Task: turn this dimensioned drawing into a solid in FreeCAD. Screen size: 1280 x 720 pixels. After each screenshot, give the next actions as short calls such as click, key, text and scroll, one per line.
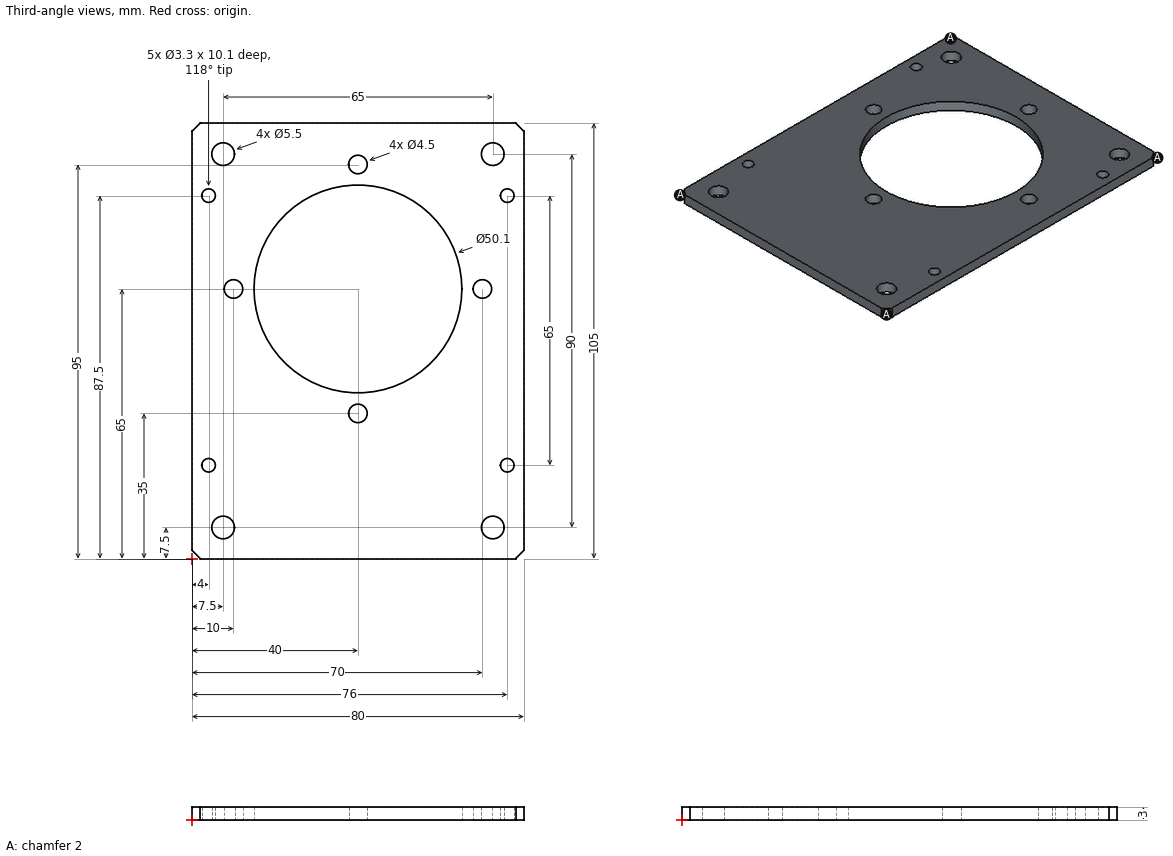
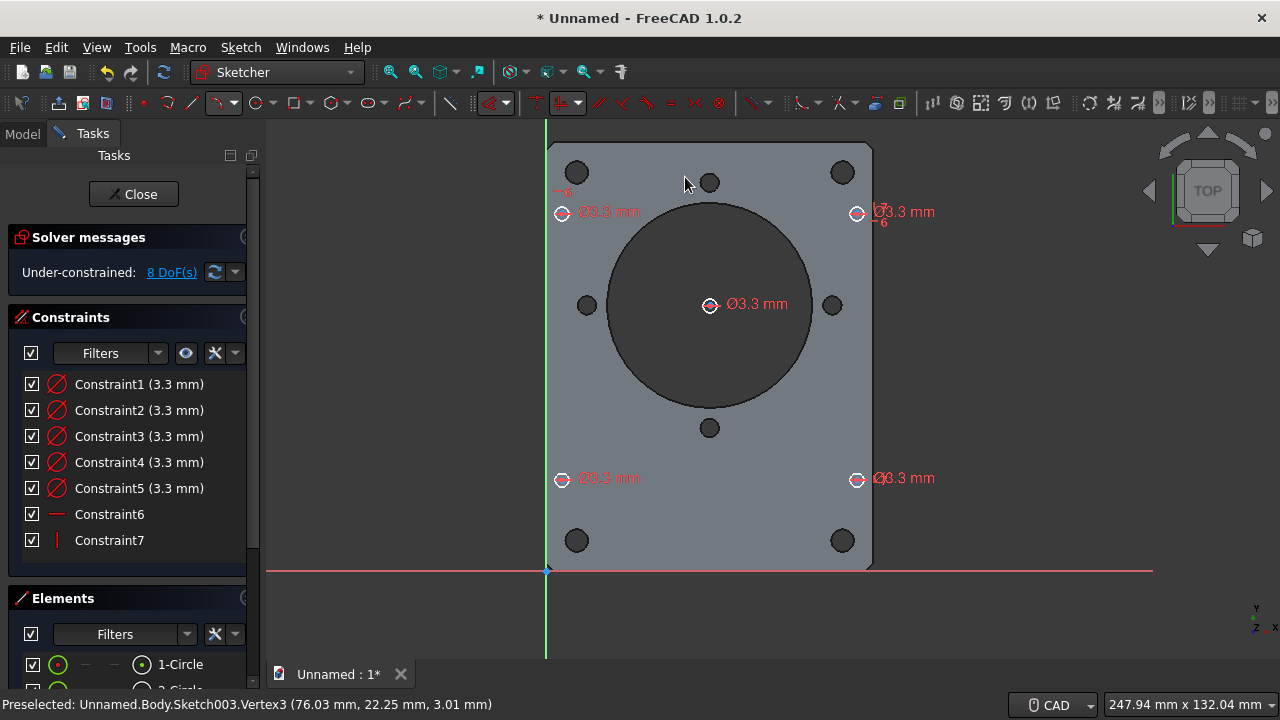
click(562, 214)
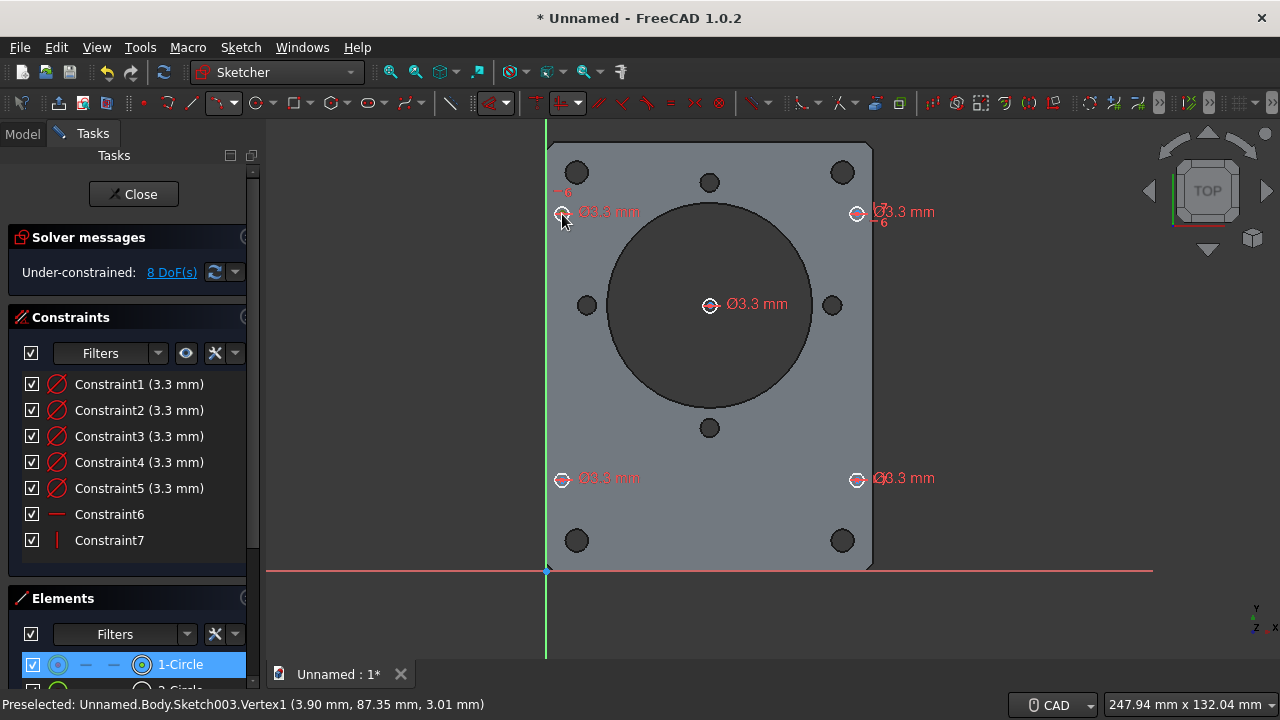
click(562, 480)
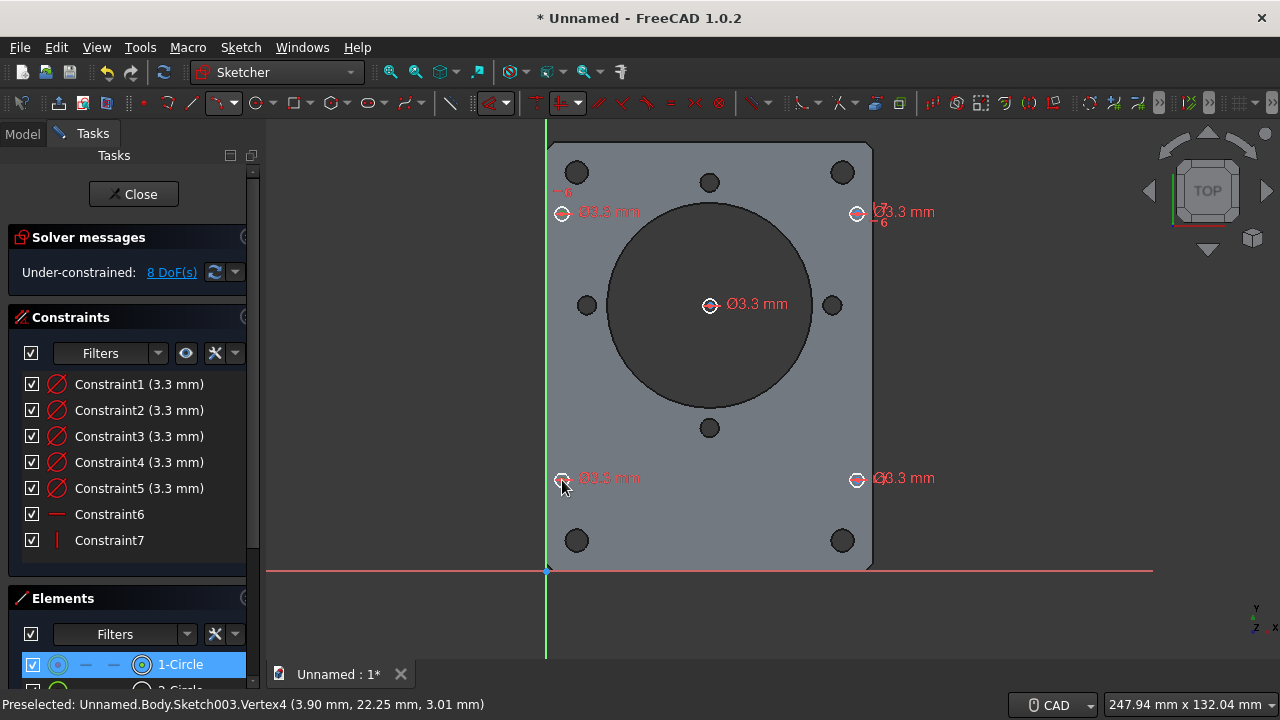
click(580, 104)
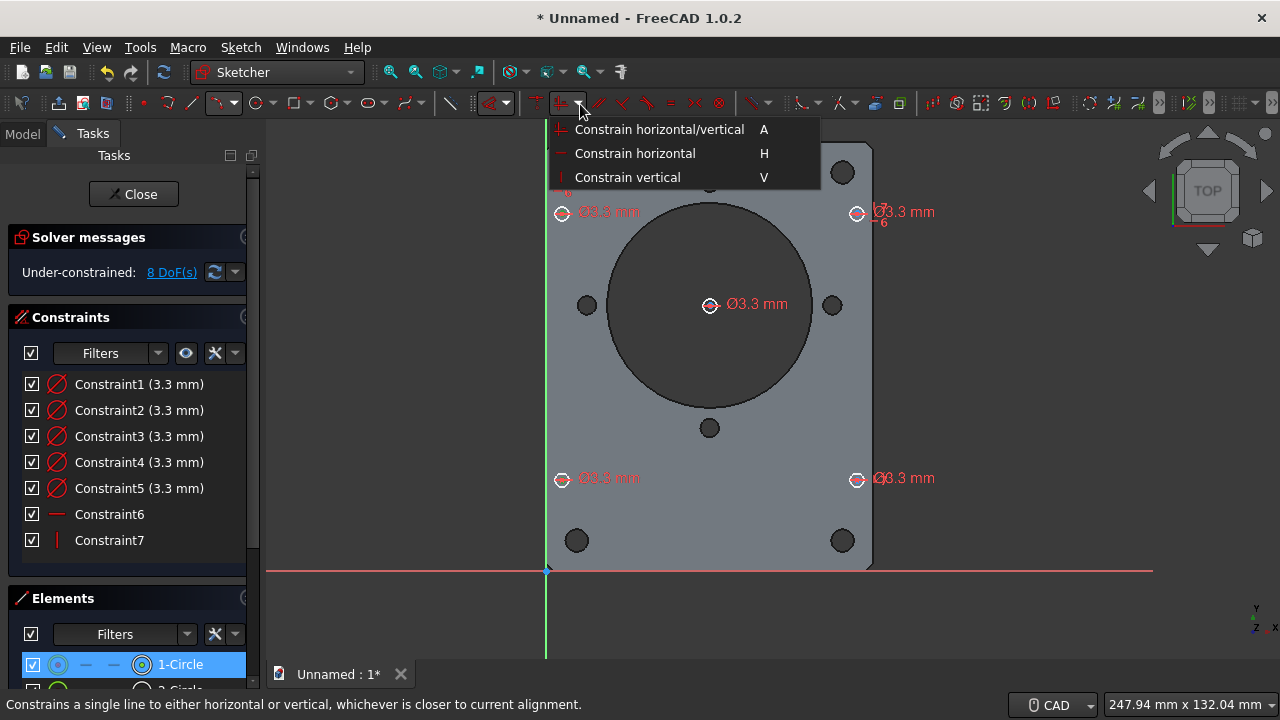
click(685, 177)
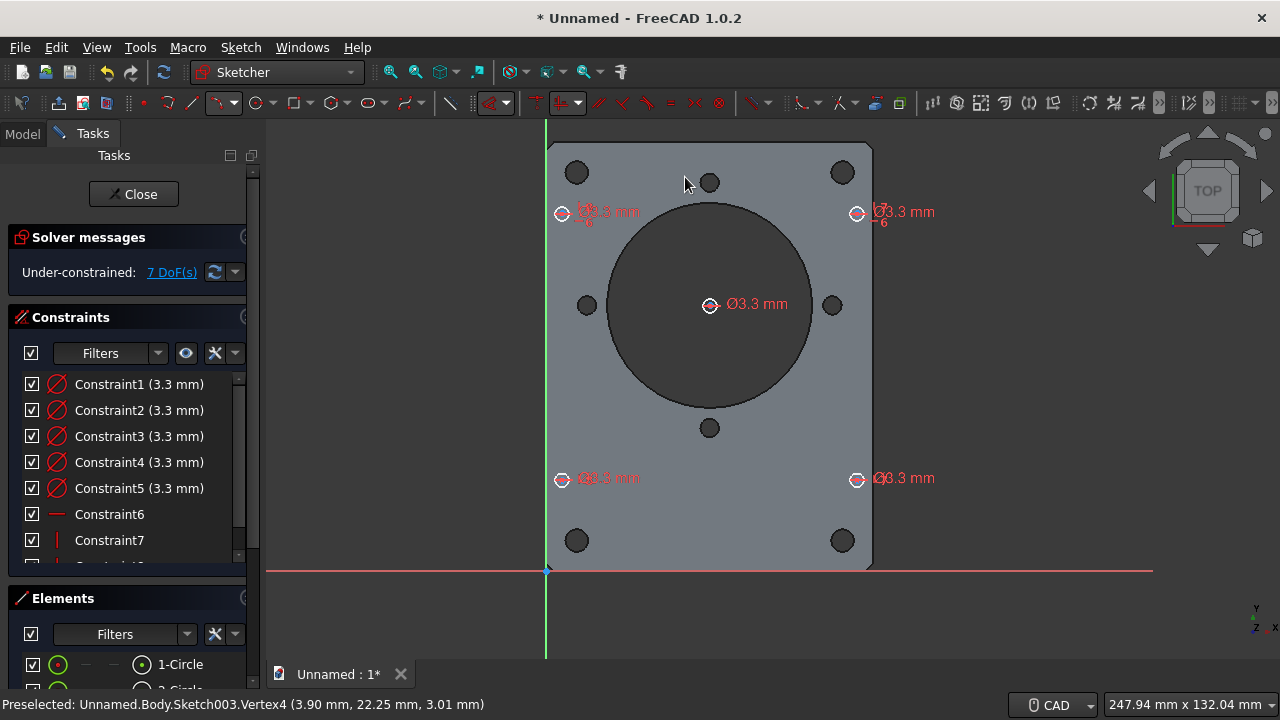
click(857, 480)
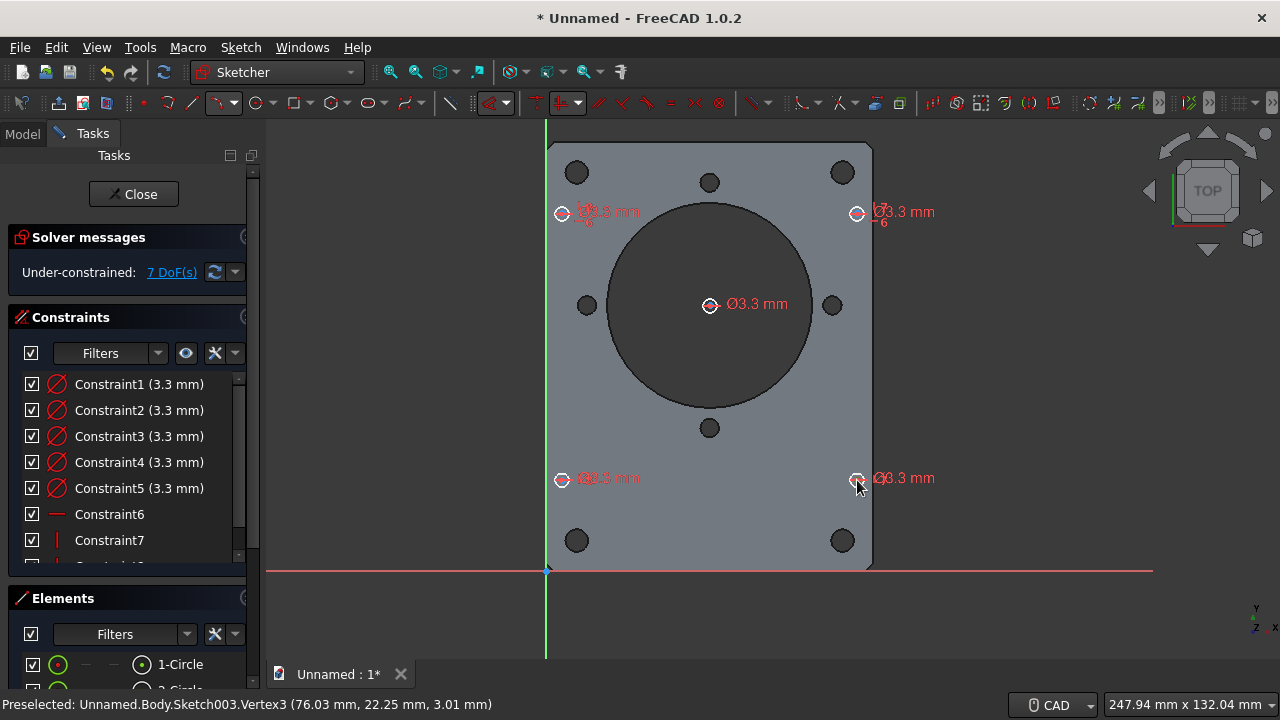
click(562, 480)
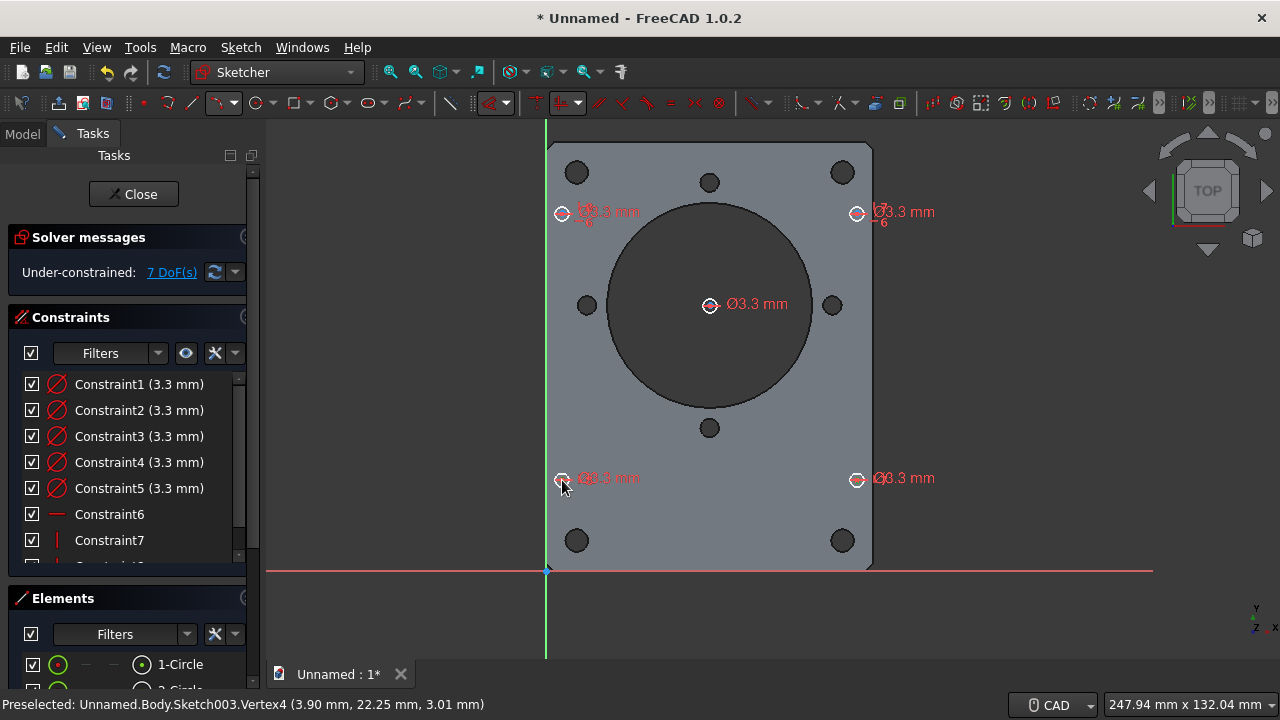
key(h)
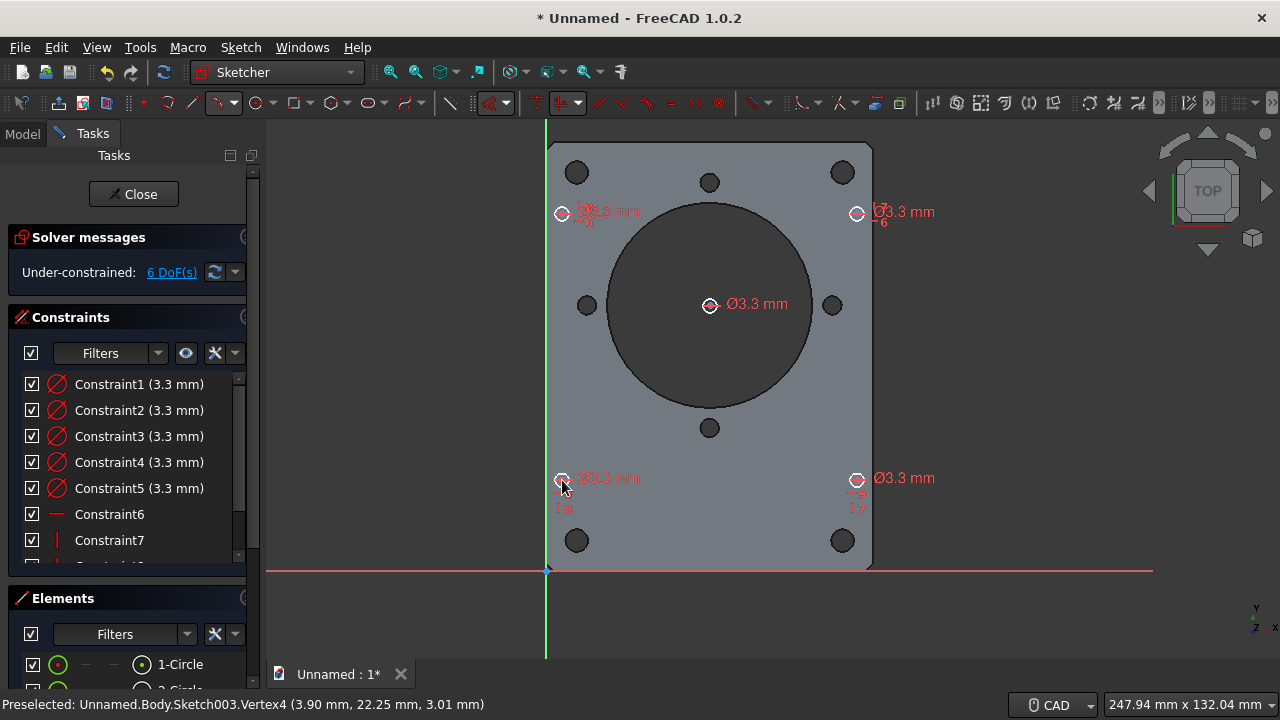
scroll(562, 214, up, 5)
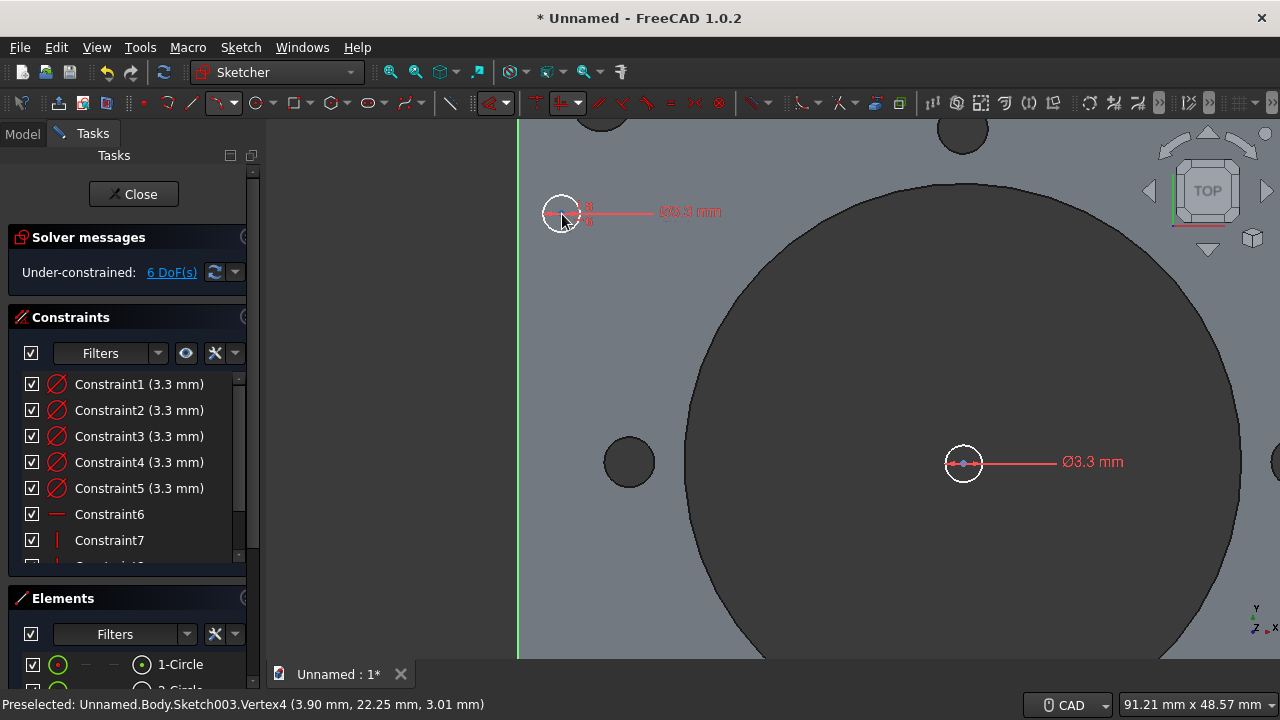
click(561, 214)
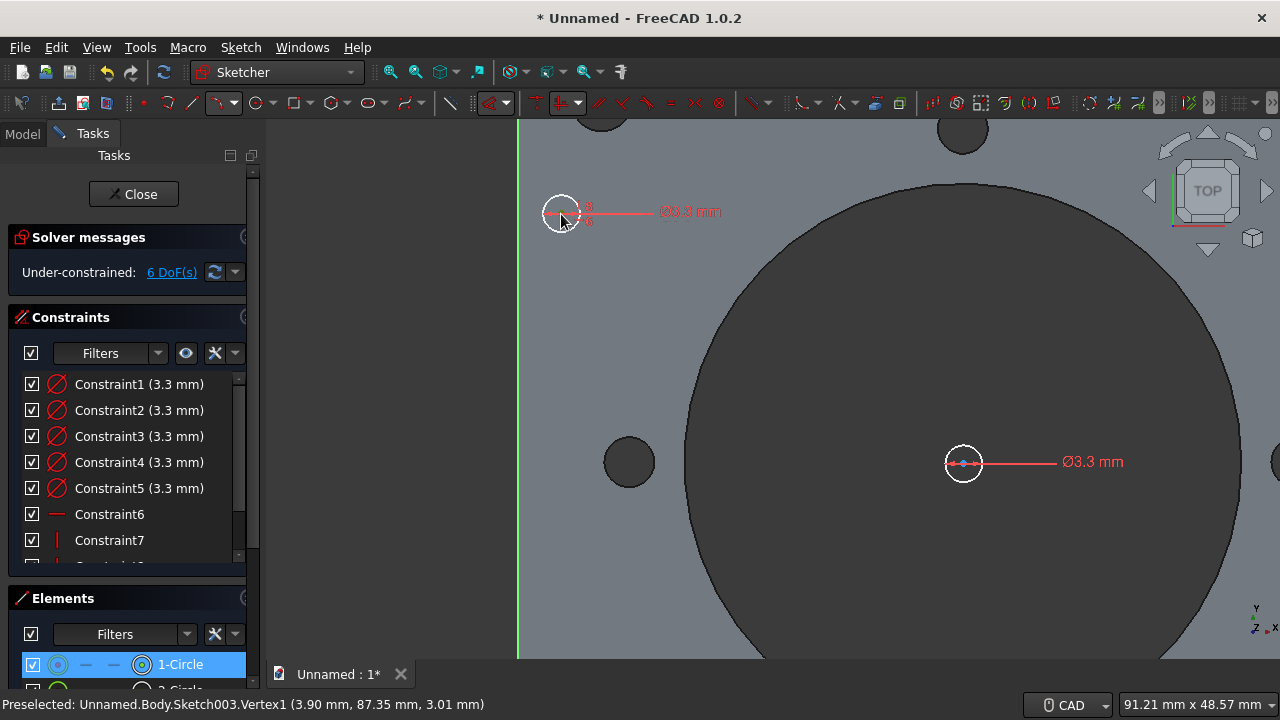
key(l)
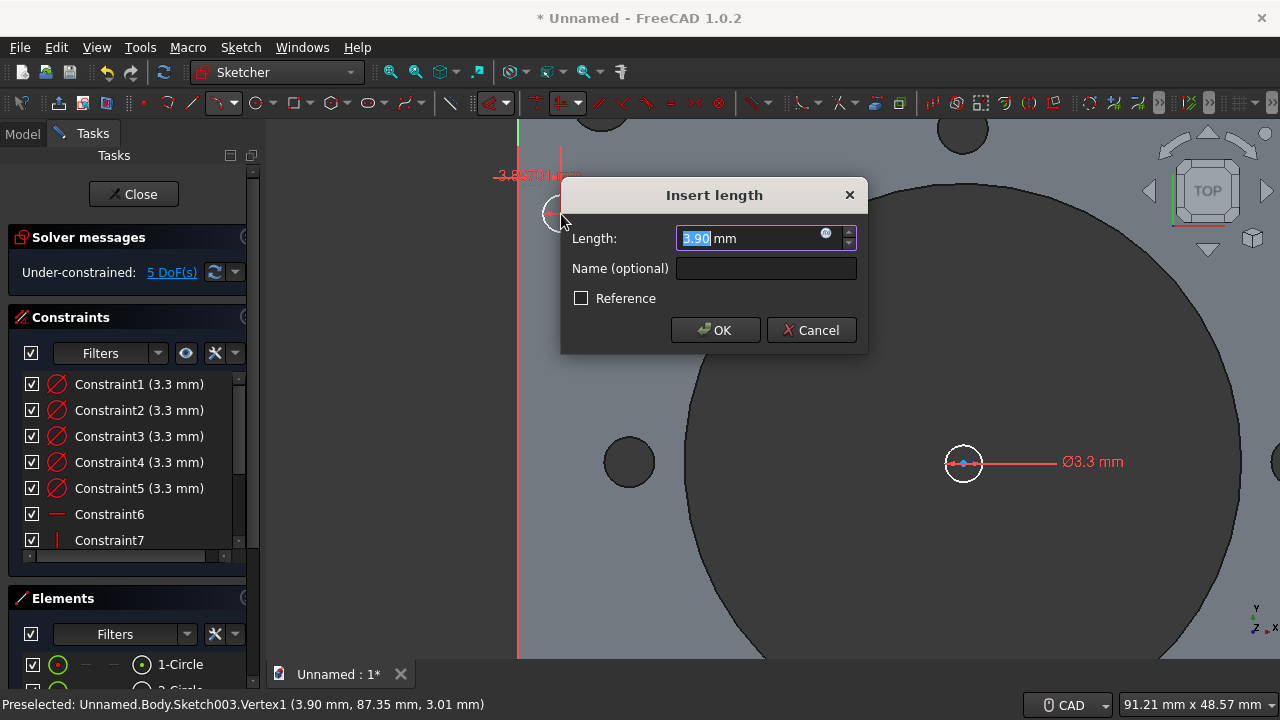
text(4)
key(Return)